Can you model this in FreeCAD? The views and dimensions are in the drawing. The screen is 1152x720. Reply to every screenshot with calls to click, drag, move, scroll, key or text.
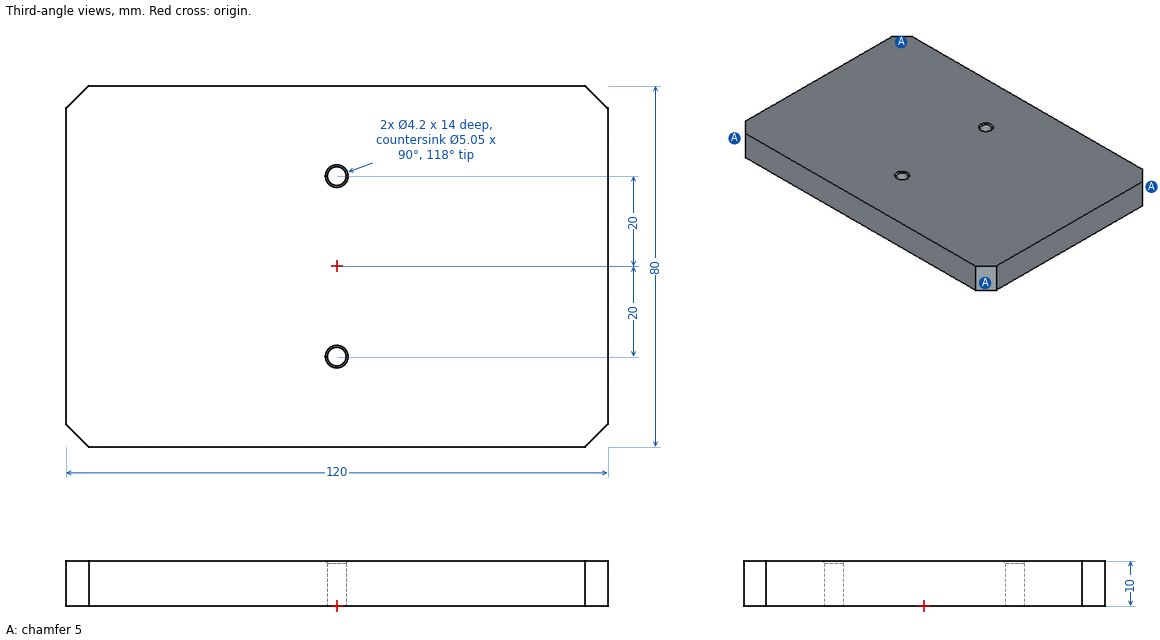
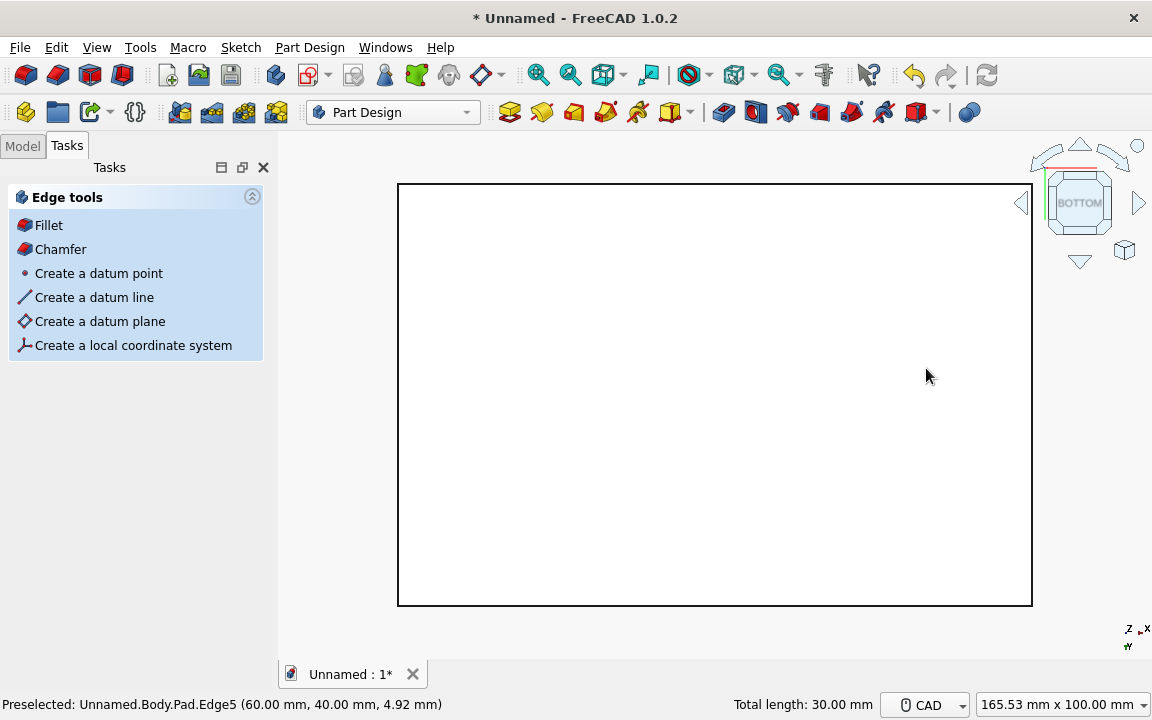
key(4)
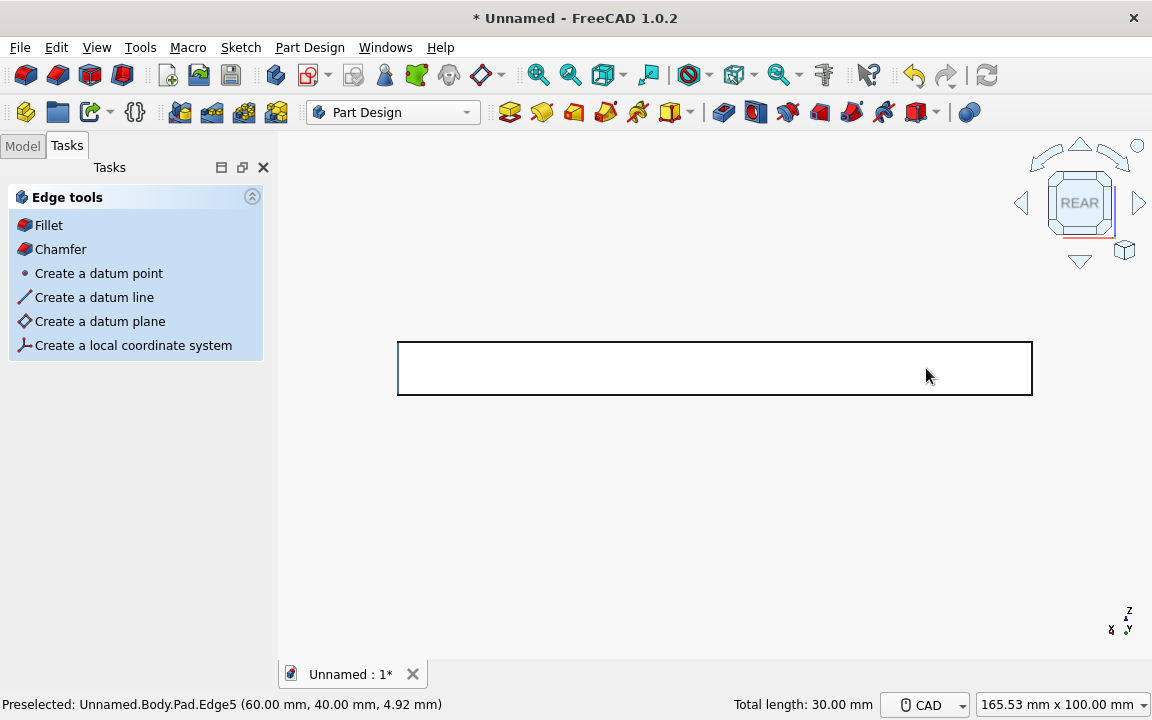
click(1032, 368, ctrl)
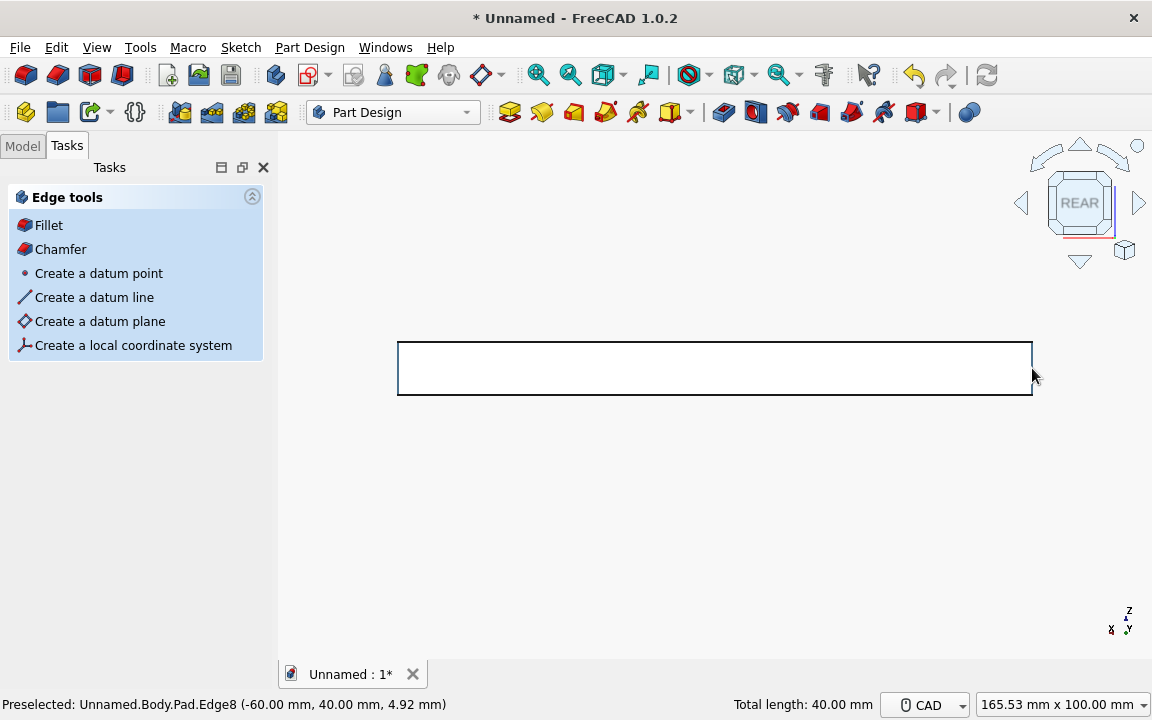
click(58, 76)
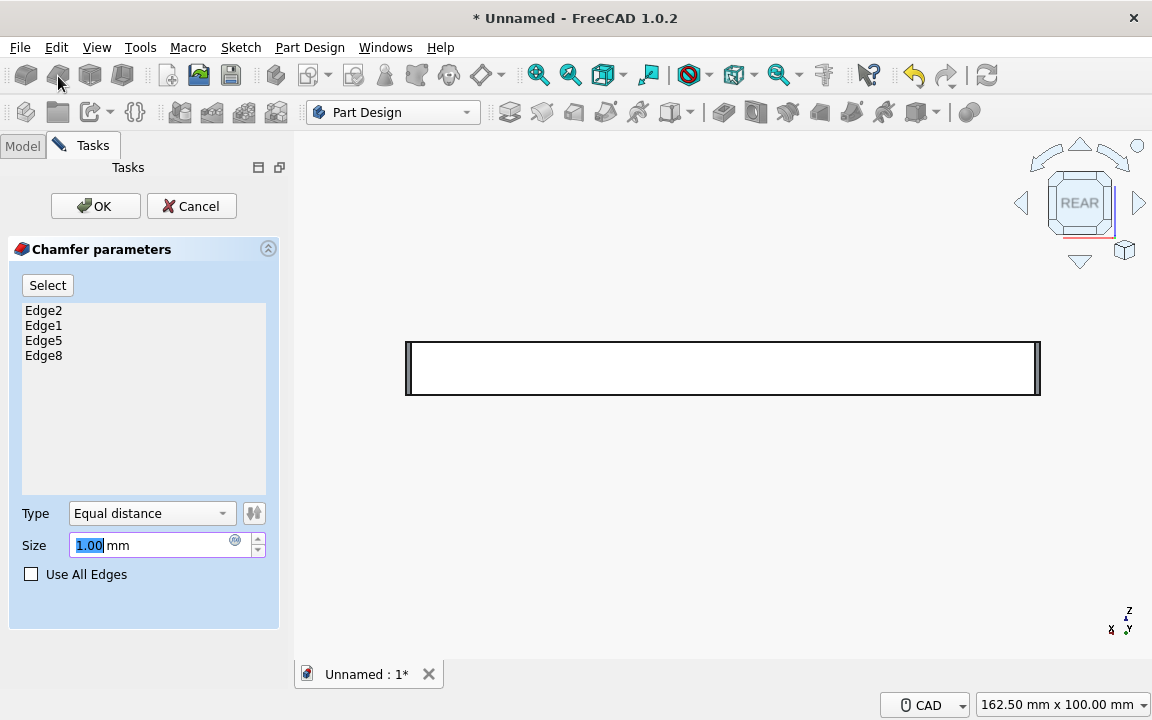
text(5)
key(Tab)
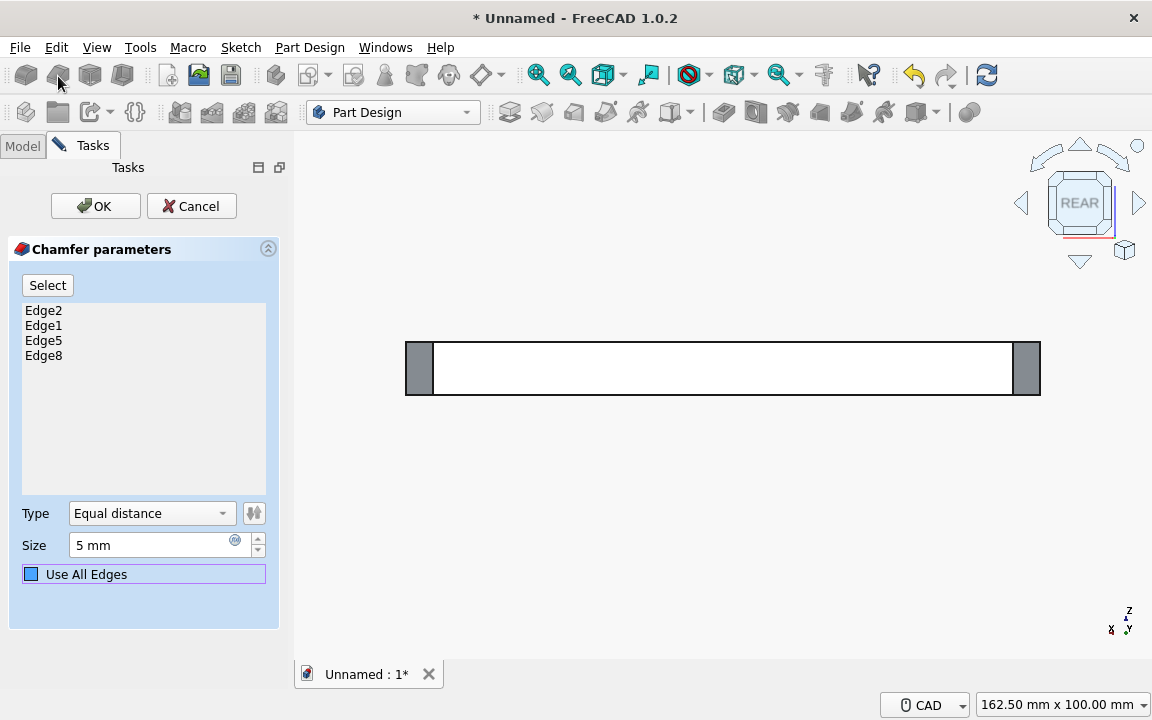
click(96, 206)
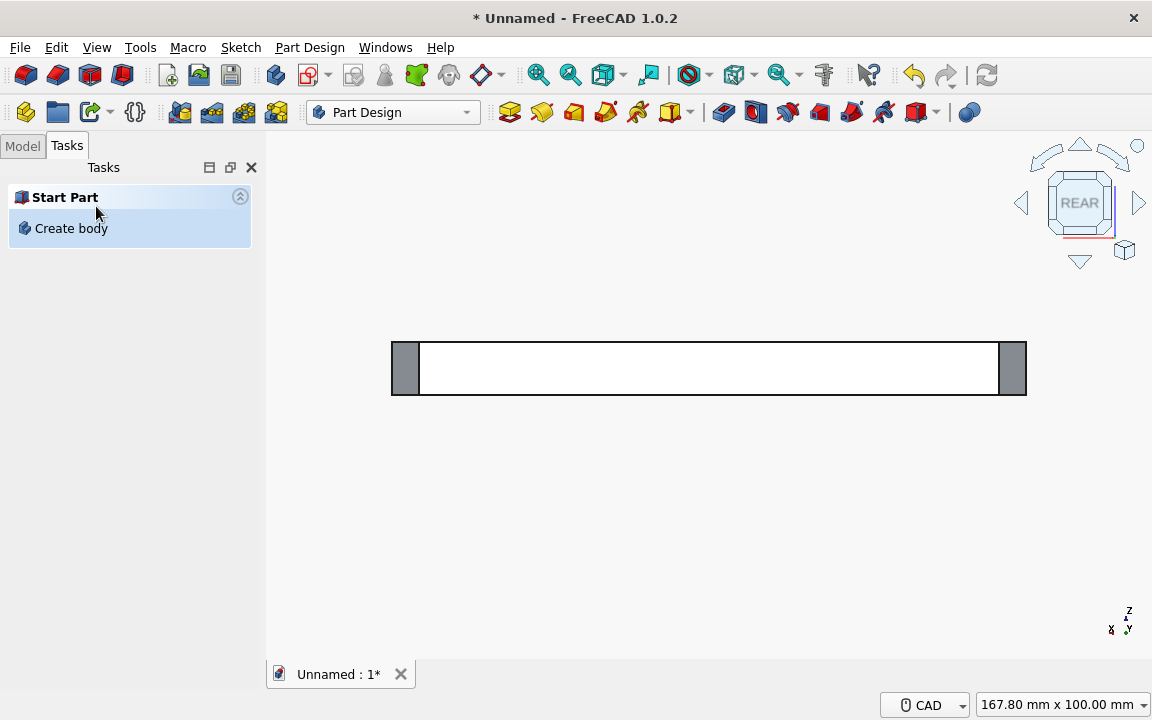
key(0)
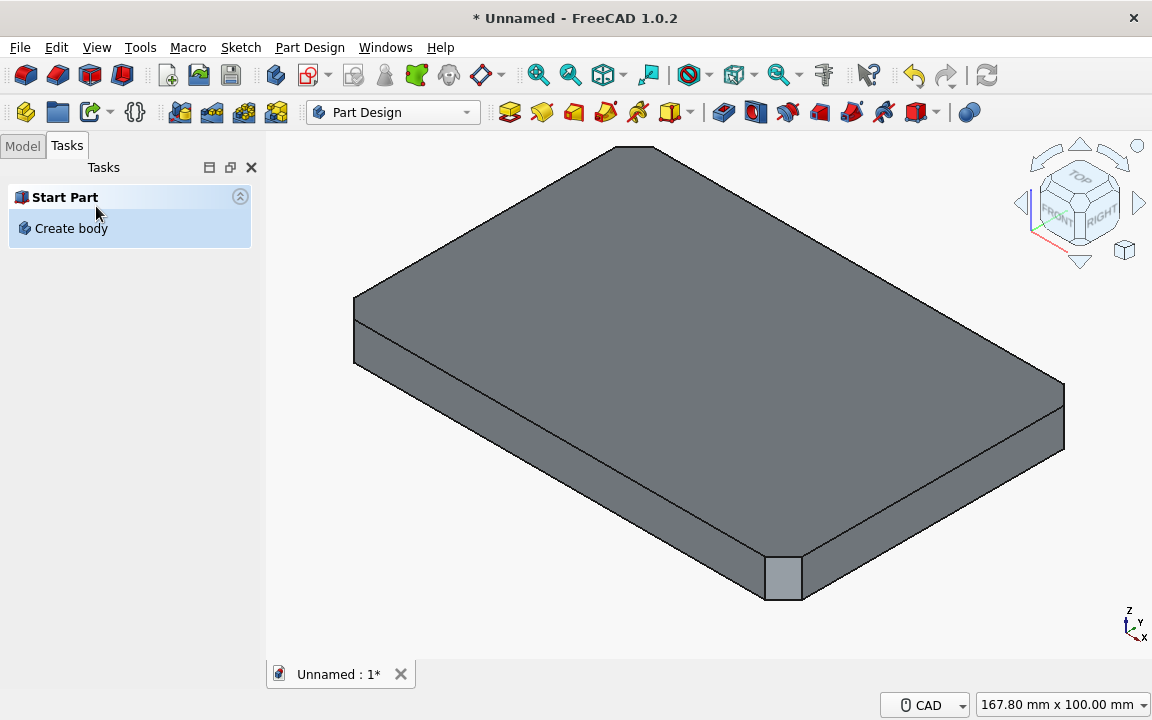
click(773, 388)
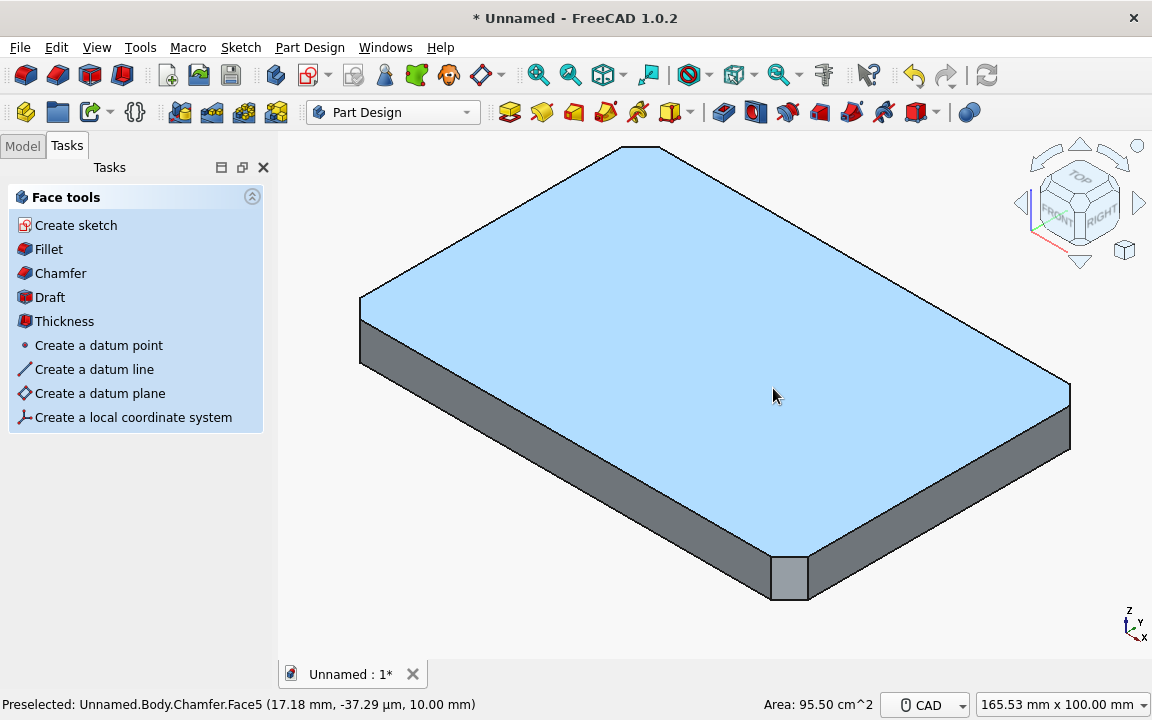
click(308, 76)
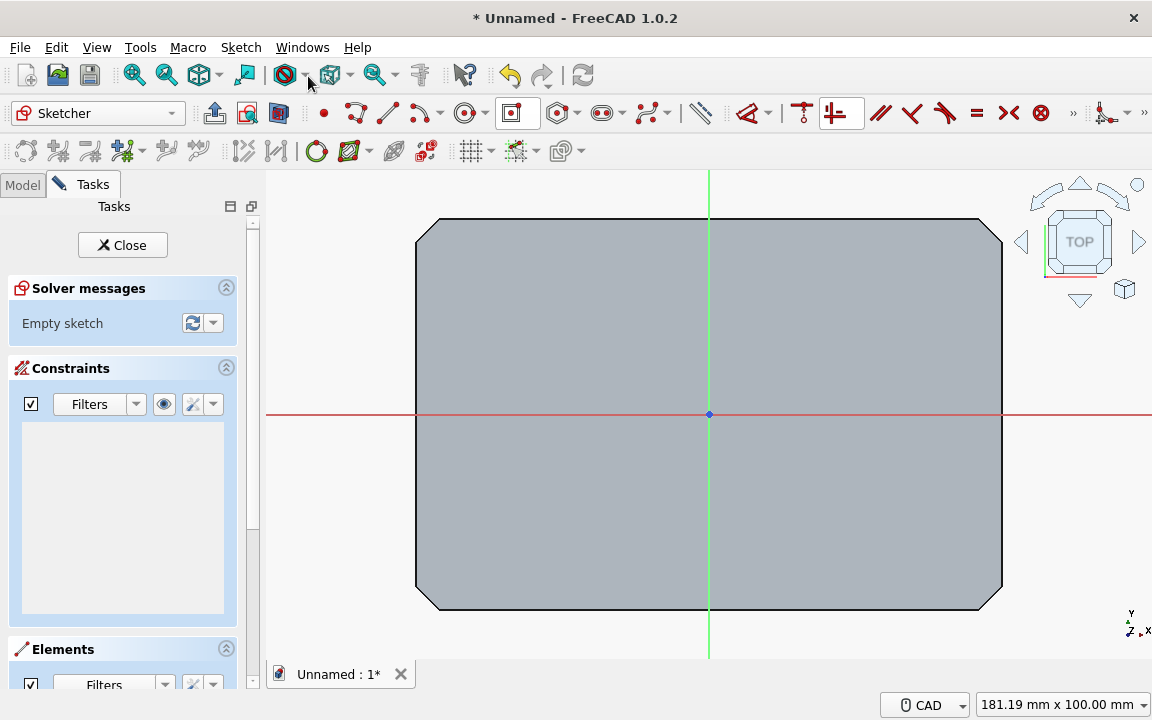
scroll(848, 414, up, 2)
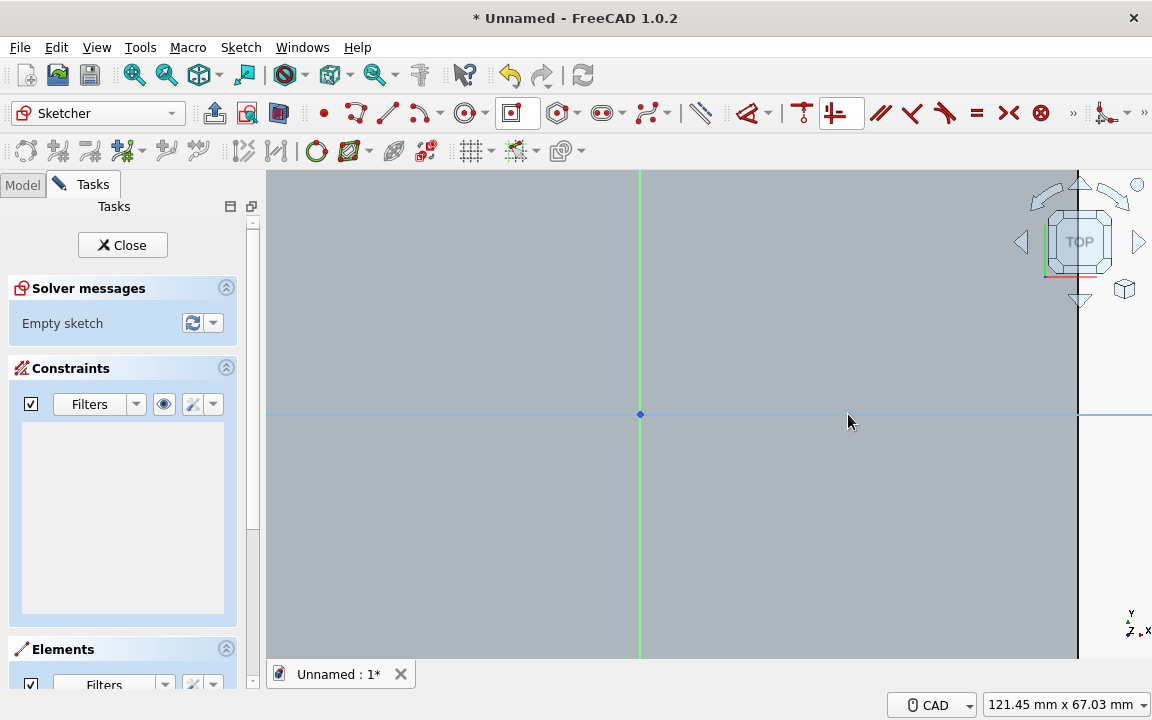
key(g)
key(c)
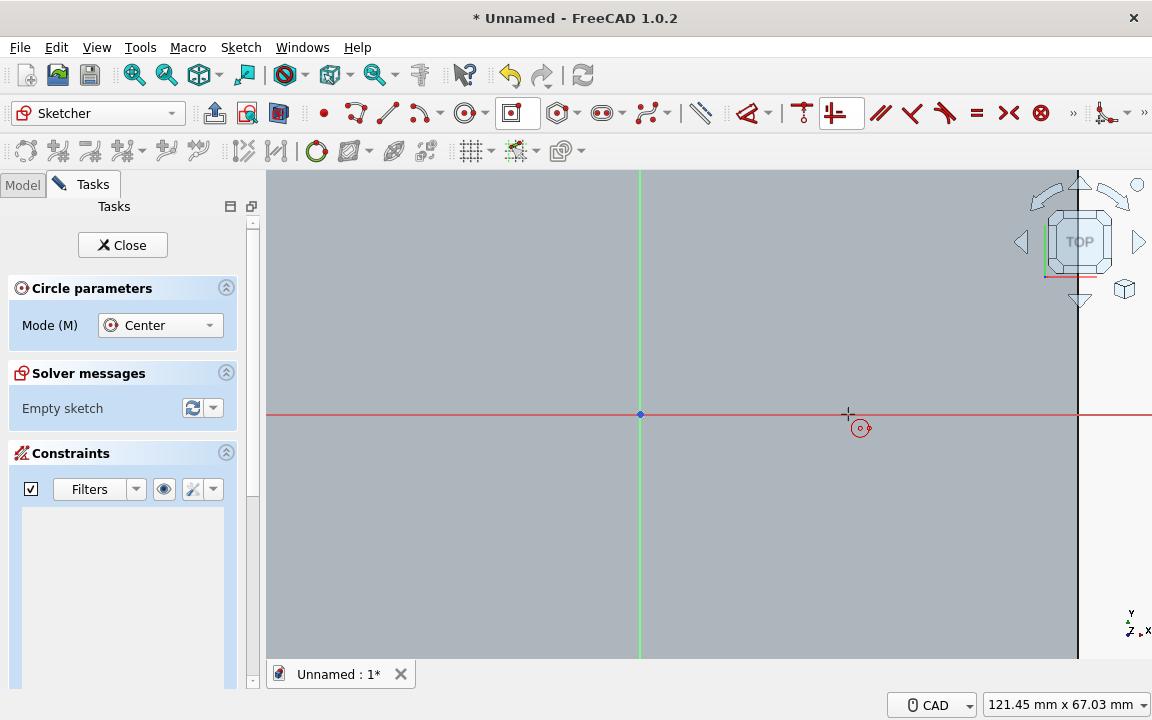
scroll(640, 269, up, 2)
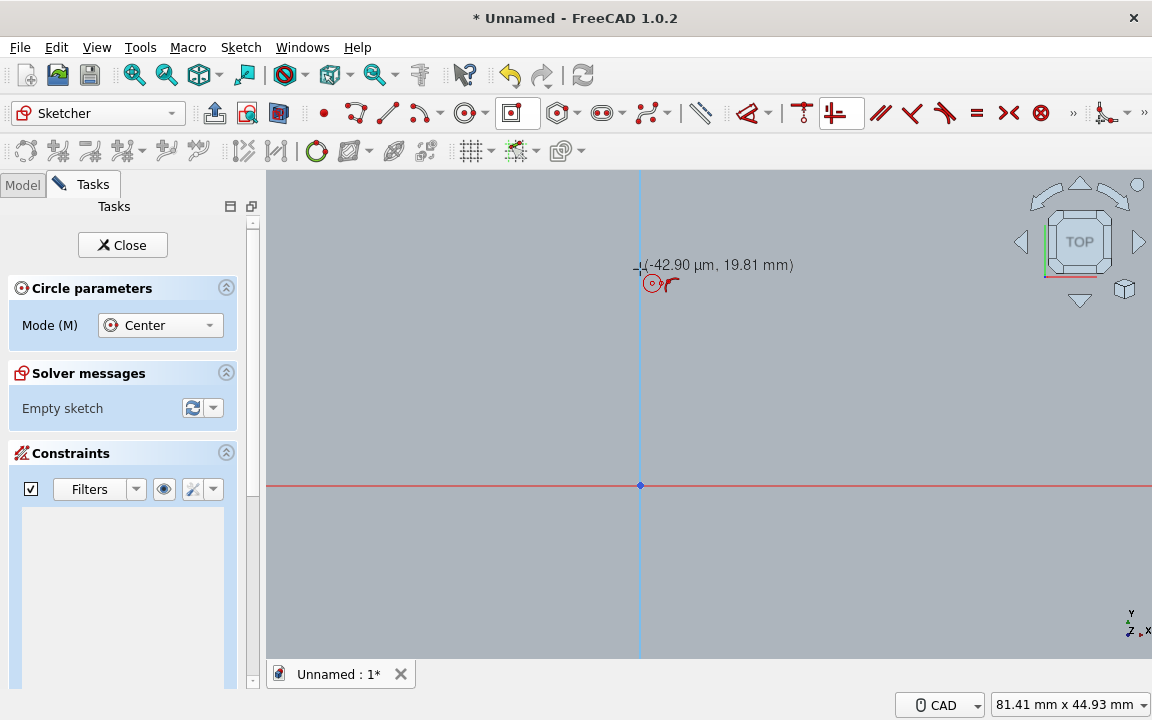
click(640, 268)
click(656, 252)